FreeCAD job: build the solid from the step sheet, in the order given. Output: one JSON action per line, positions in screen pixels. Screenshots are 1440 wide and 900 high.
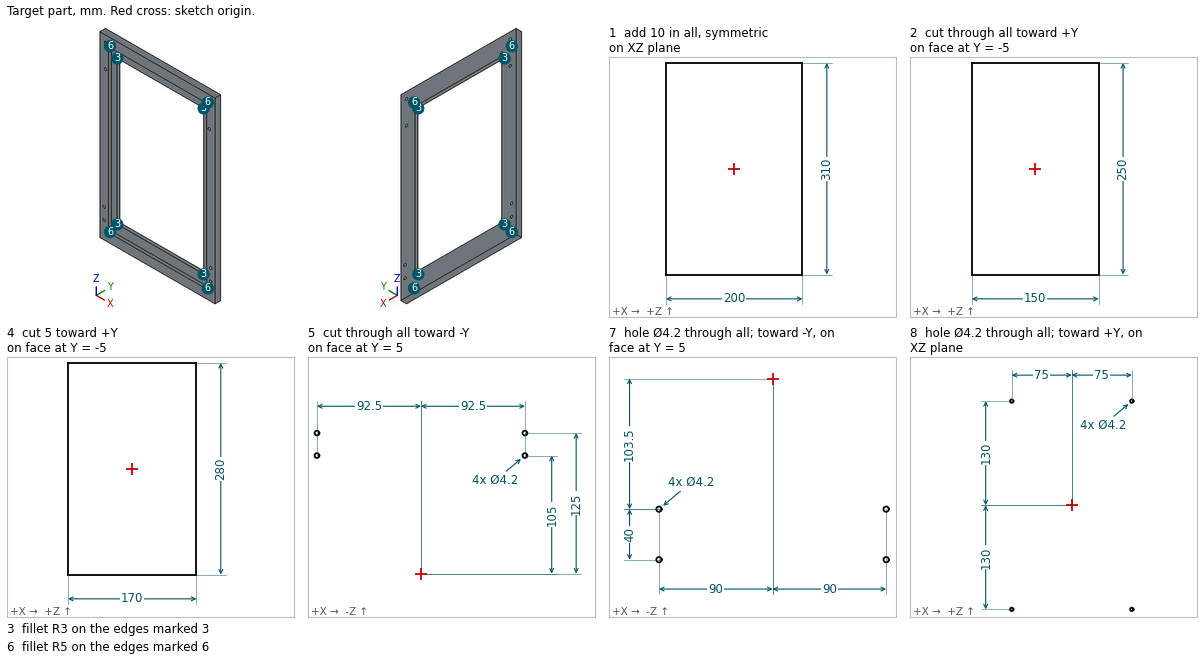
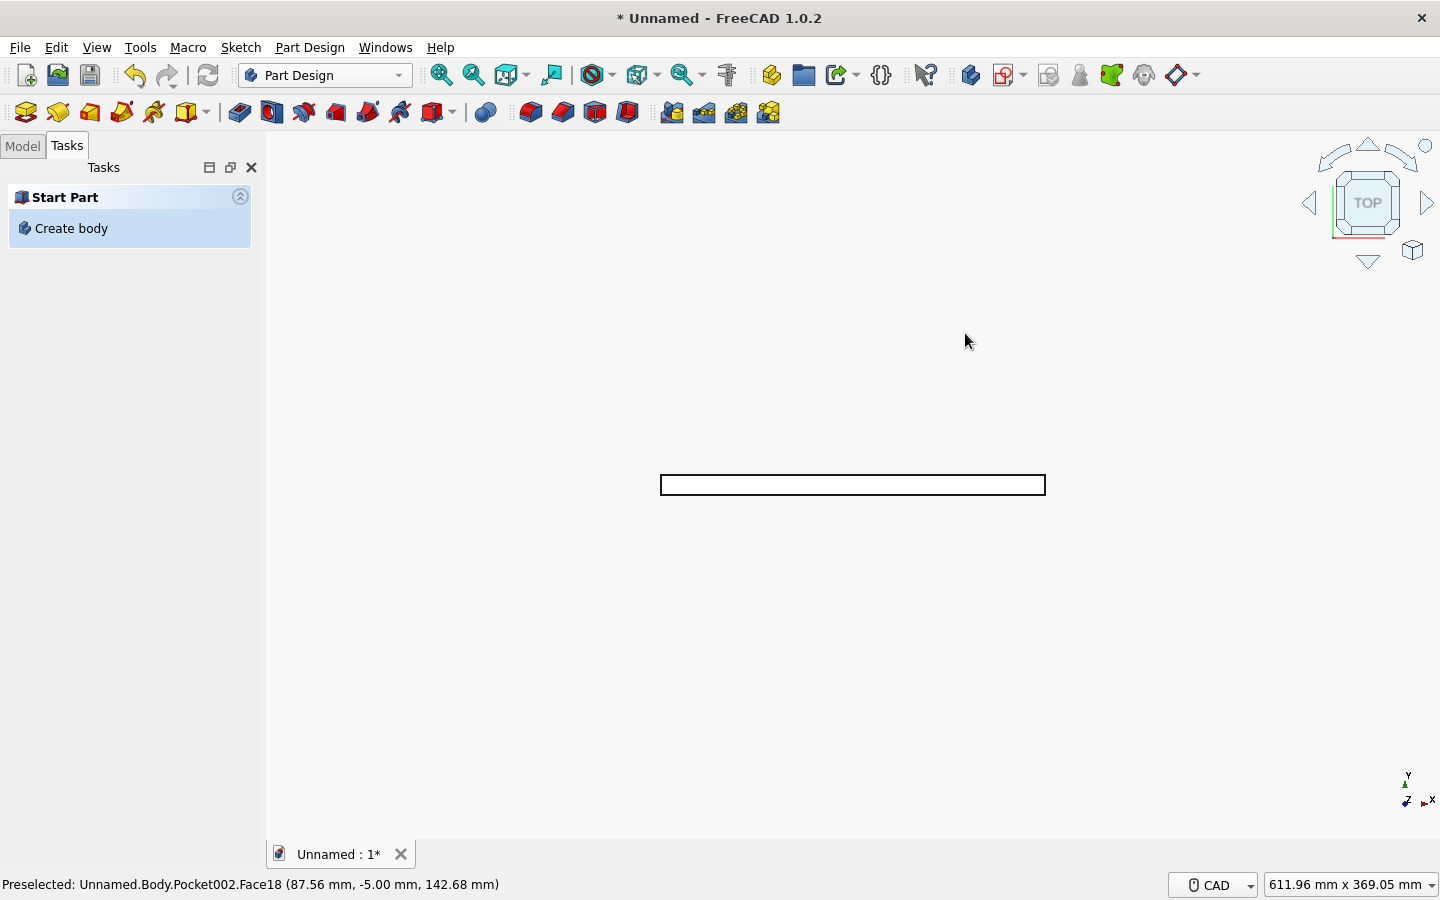
{"action": "left_click", "coordinate": [442, 76]}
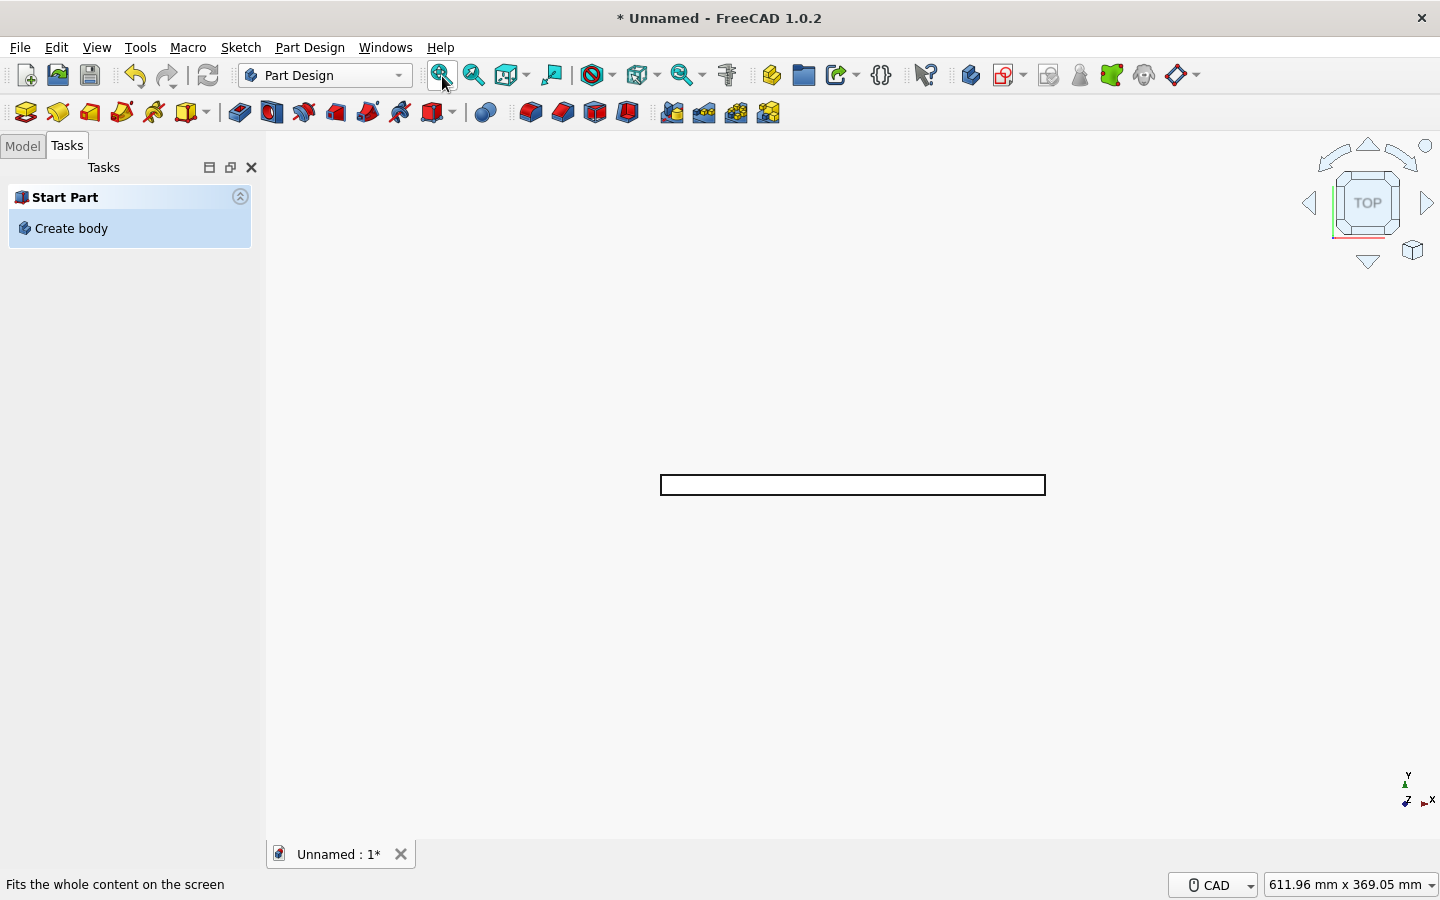
{"action": "scroll", "coordinate": [1016, 489], "scroll_direction": "up", "scroll_amount": 8}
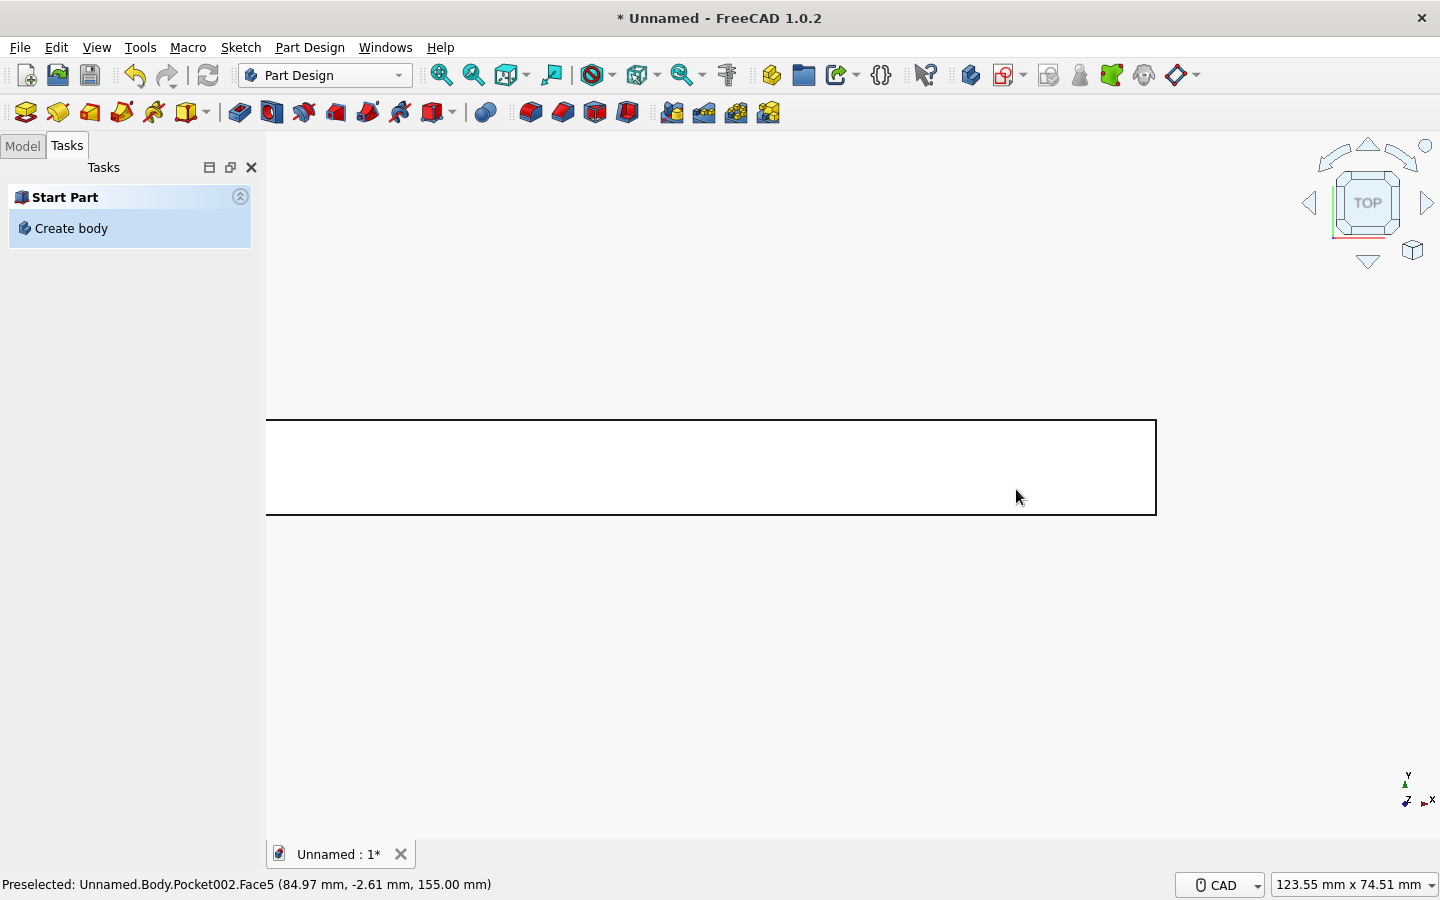
{"action": "key", "text": "v f"}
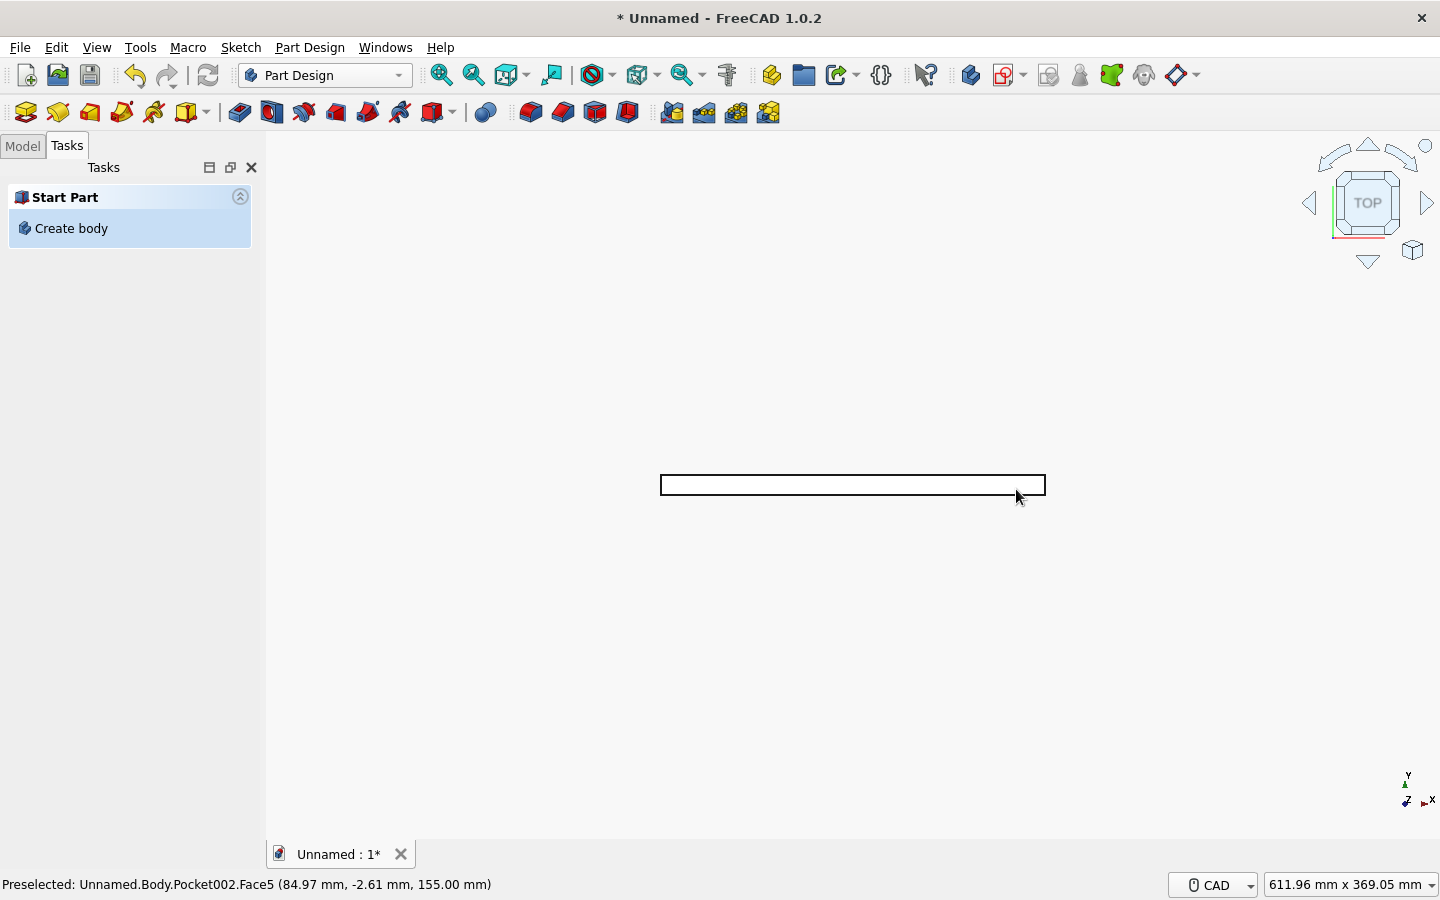
{"action": "key", "text": "1"}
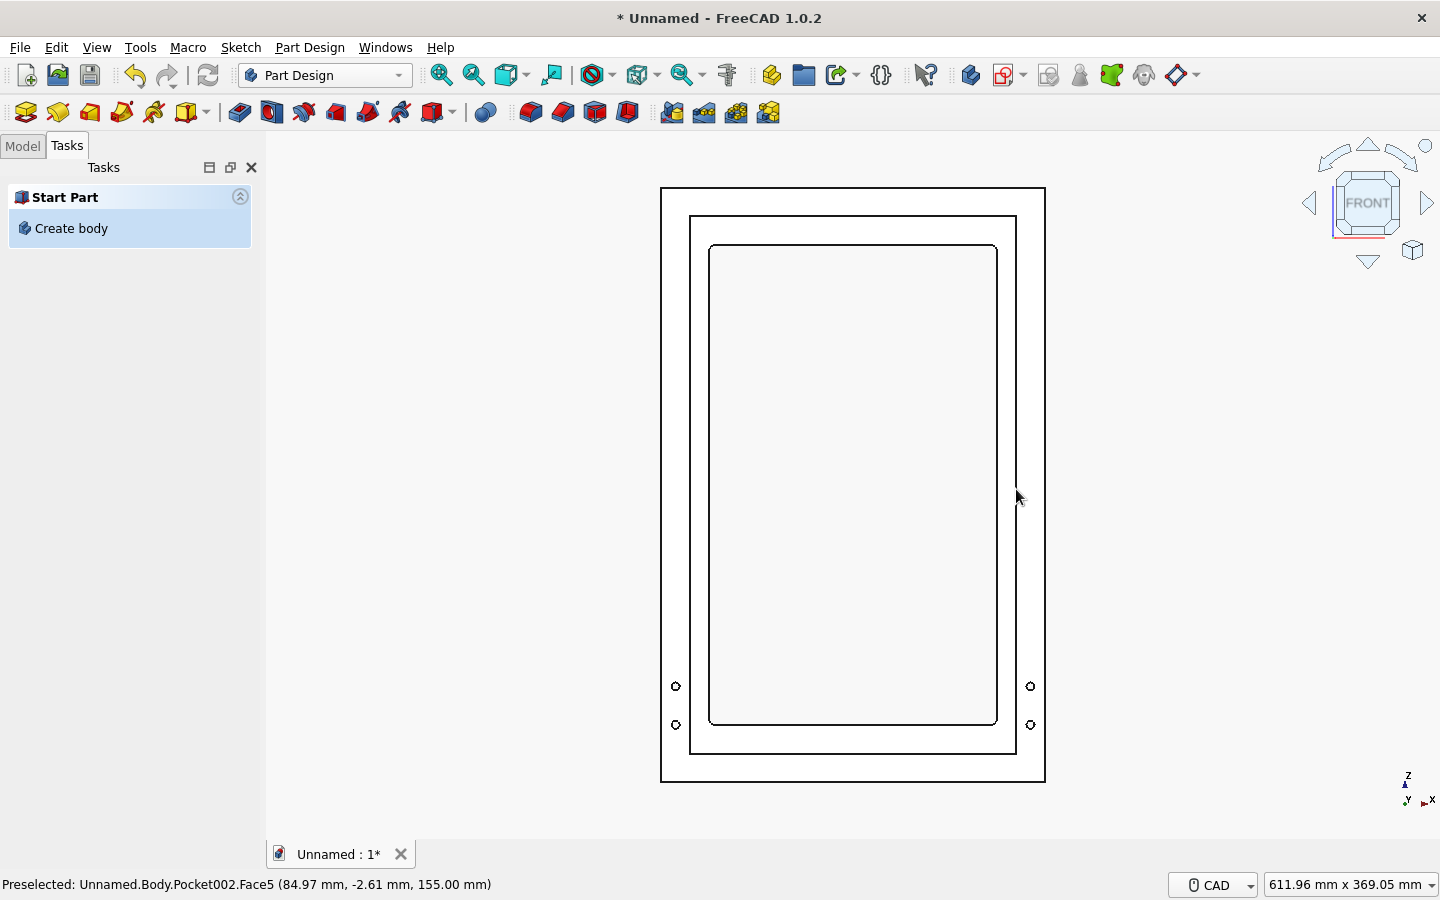
{"action": "scroll", "coordinate": [1016, 215], "scroll_direction": "up", "scroll_amount": 8}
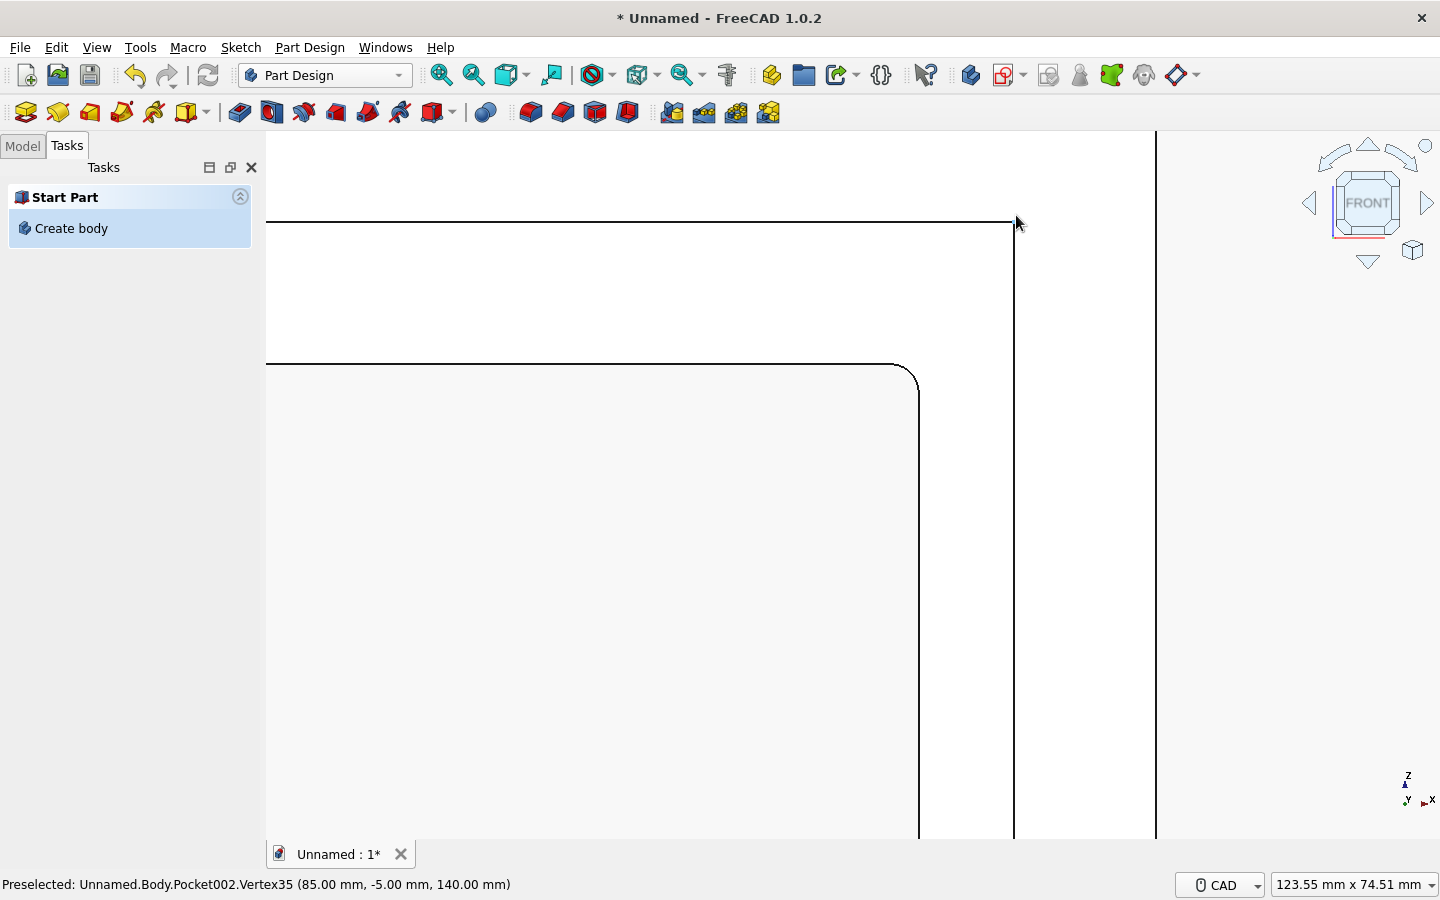
{"action": "left_click", "coordinate": [442, 76]}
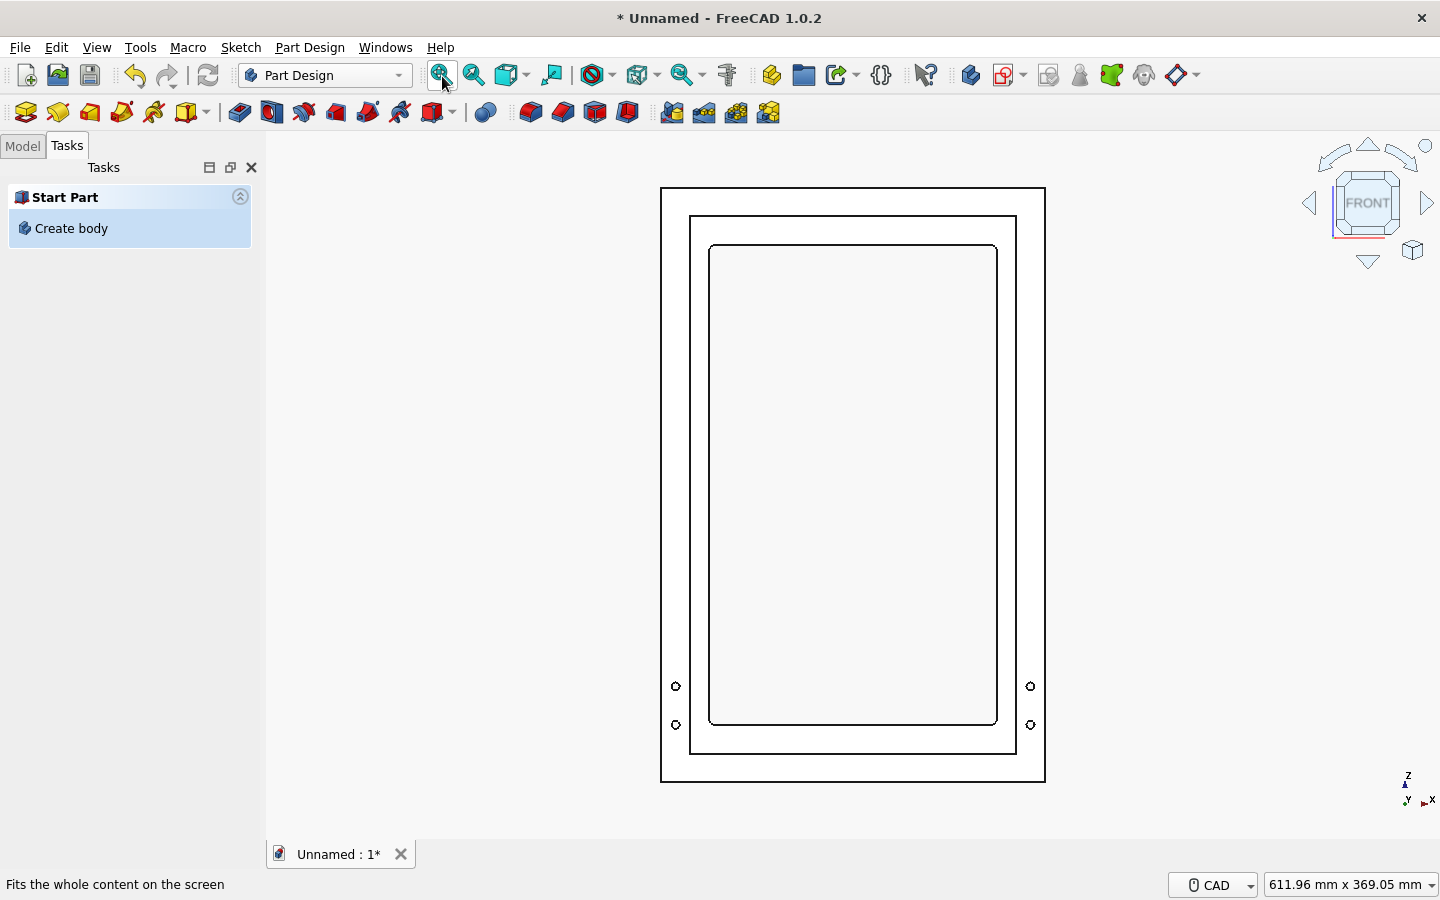
{"action": "key", "text": "3"}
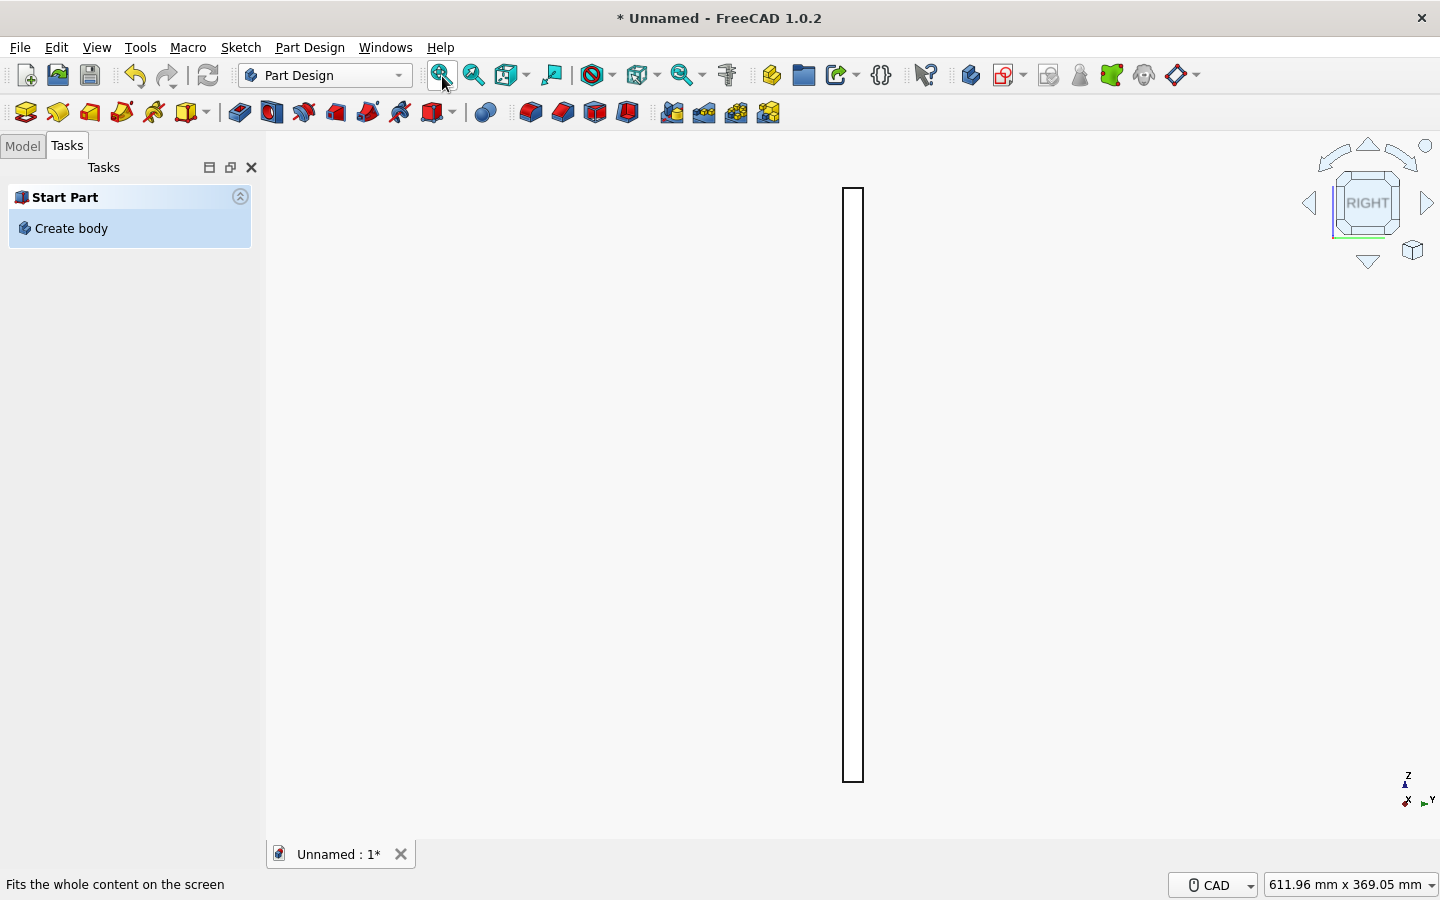
{"action": "scroll", "coordinate": [848, 215], "scroll_direction": "up", "scroll_amount": 8}